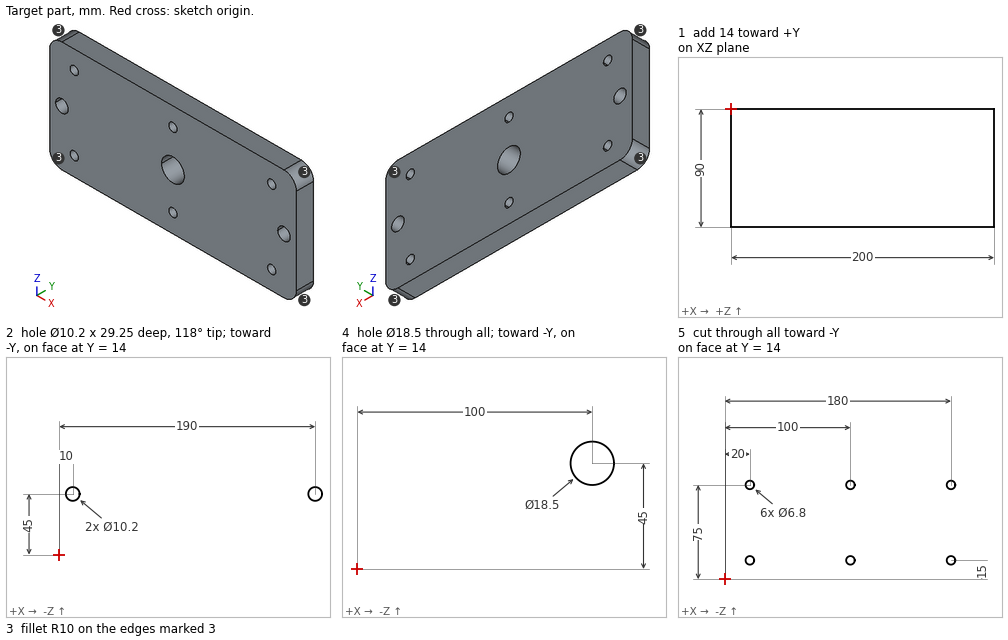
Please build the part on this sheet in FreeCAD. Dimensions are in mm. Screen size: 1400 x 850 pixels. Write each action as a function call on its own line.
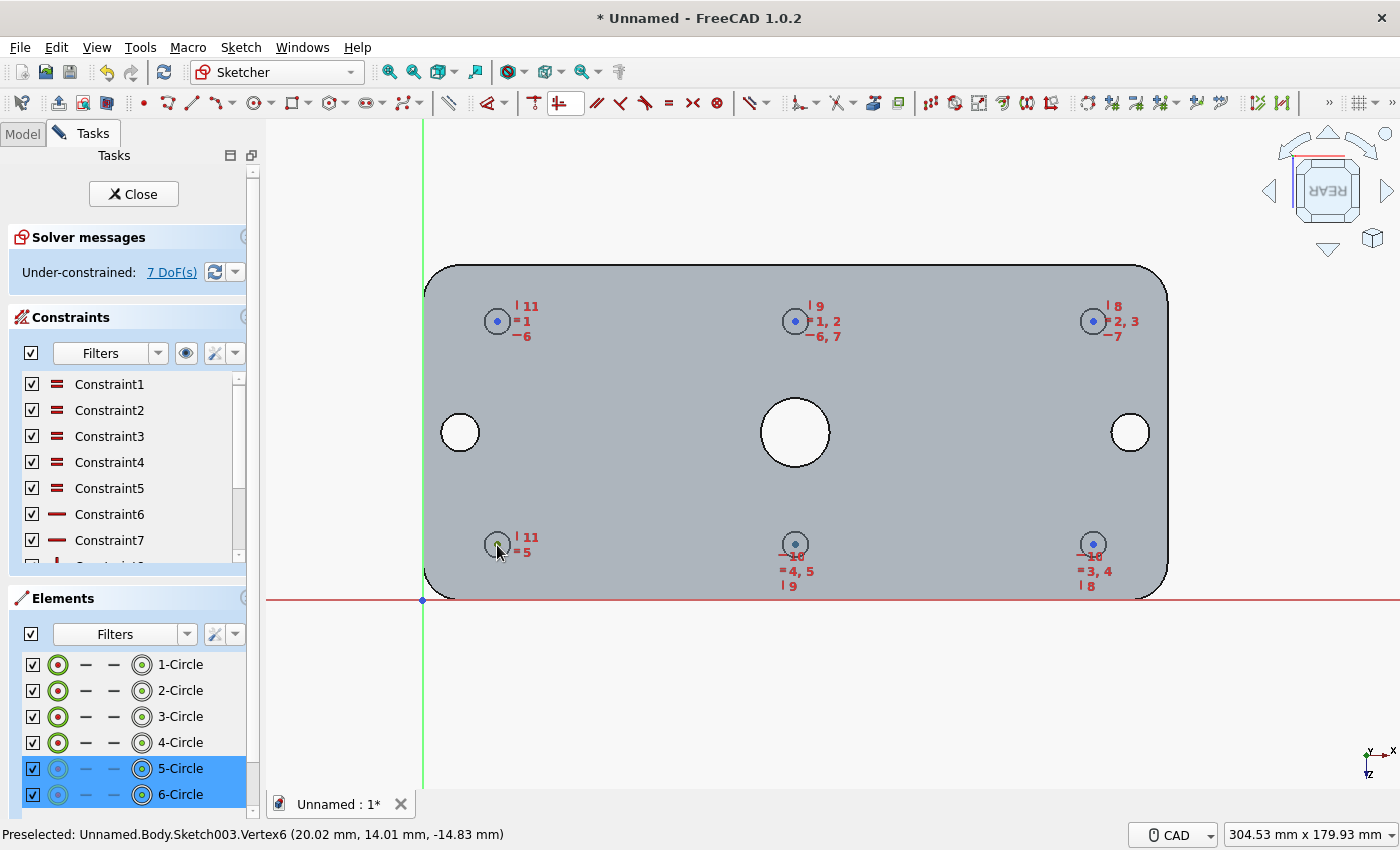
click(578, 104)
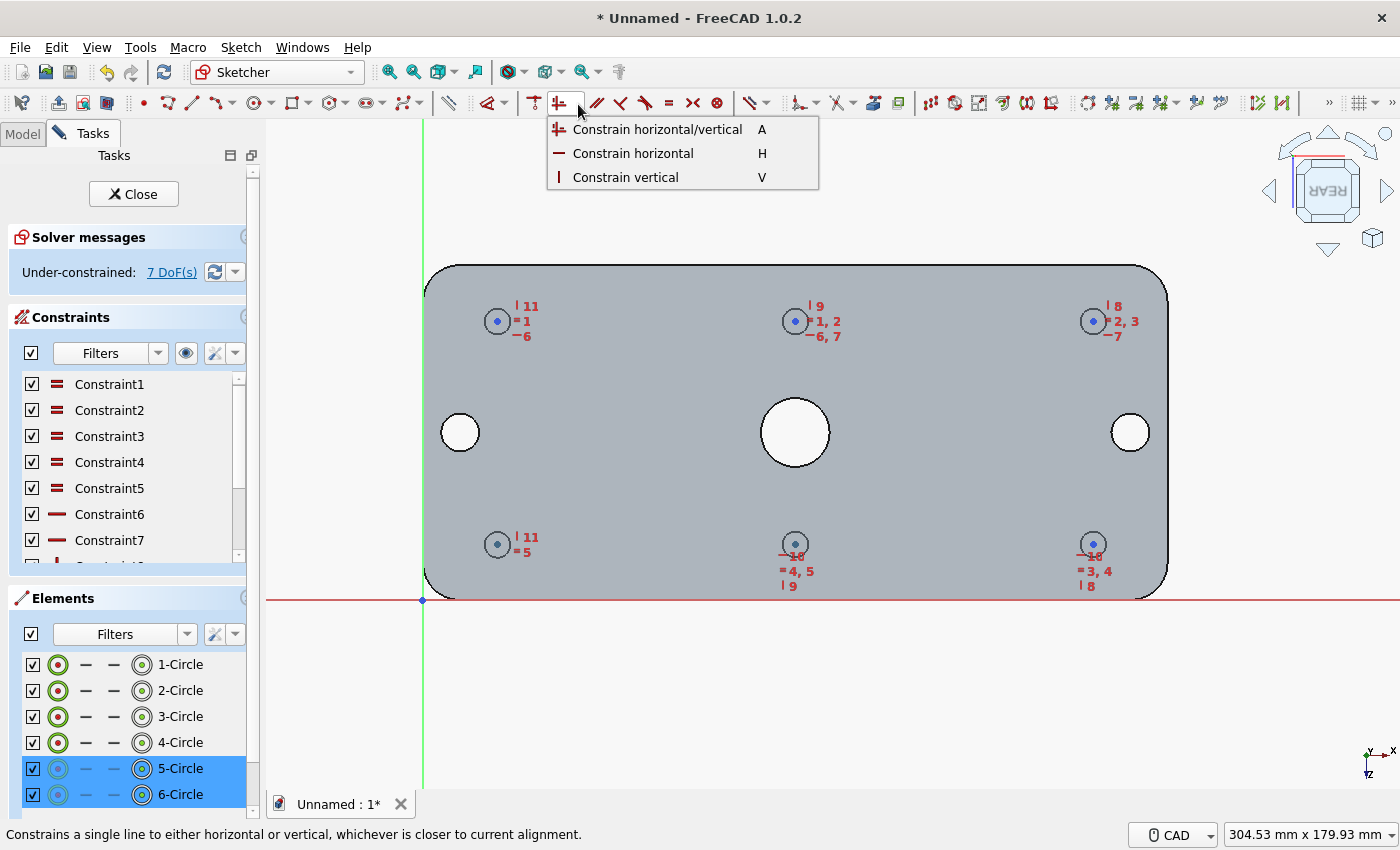
click(683, 153)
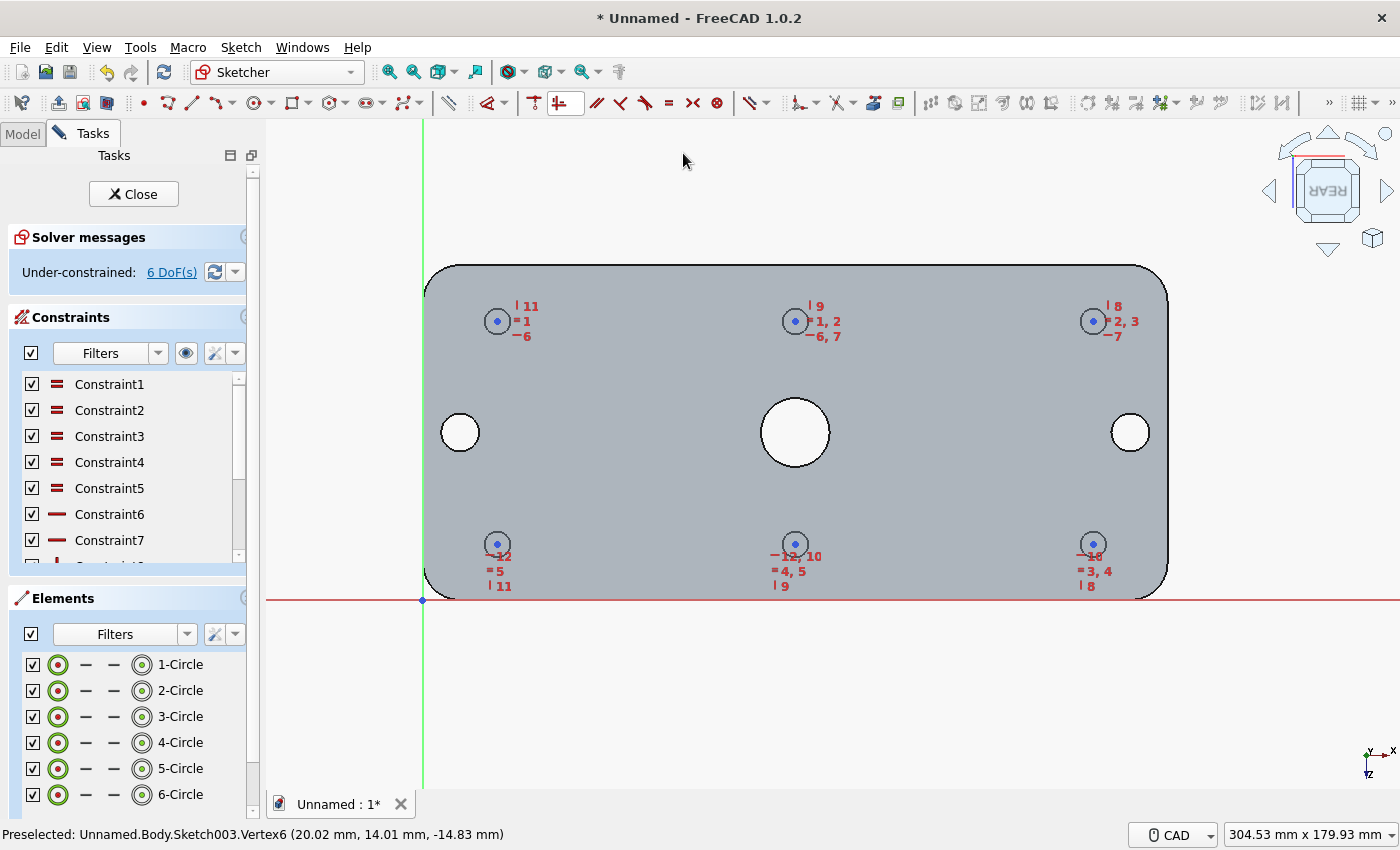
key(d)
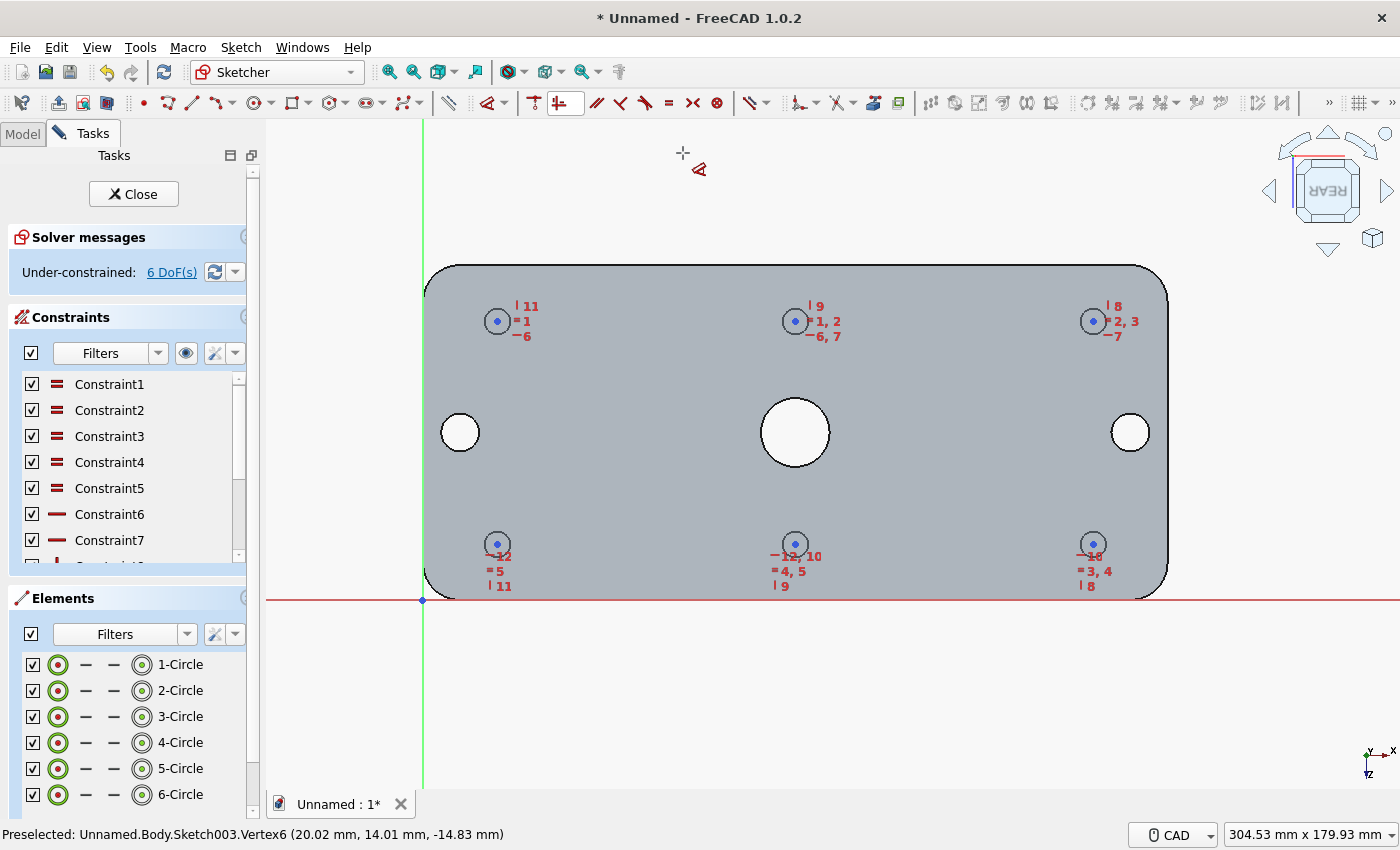
scroll(506, 313, up, 3)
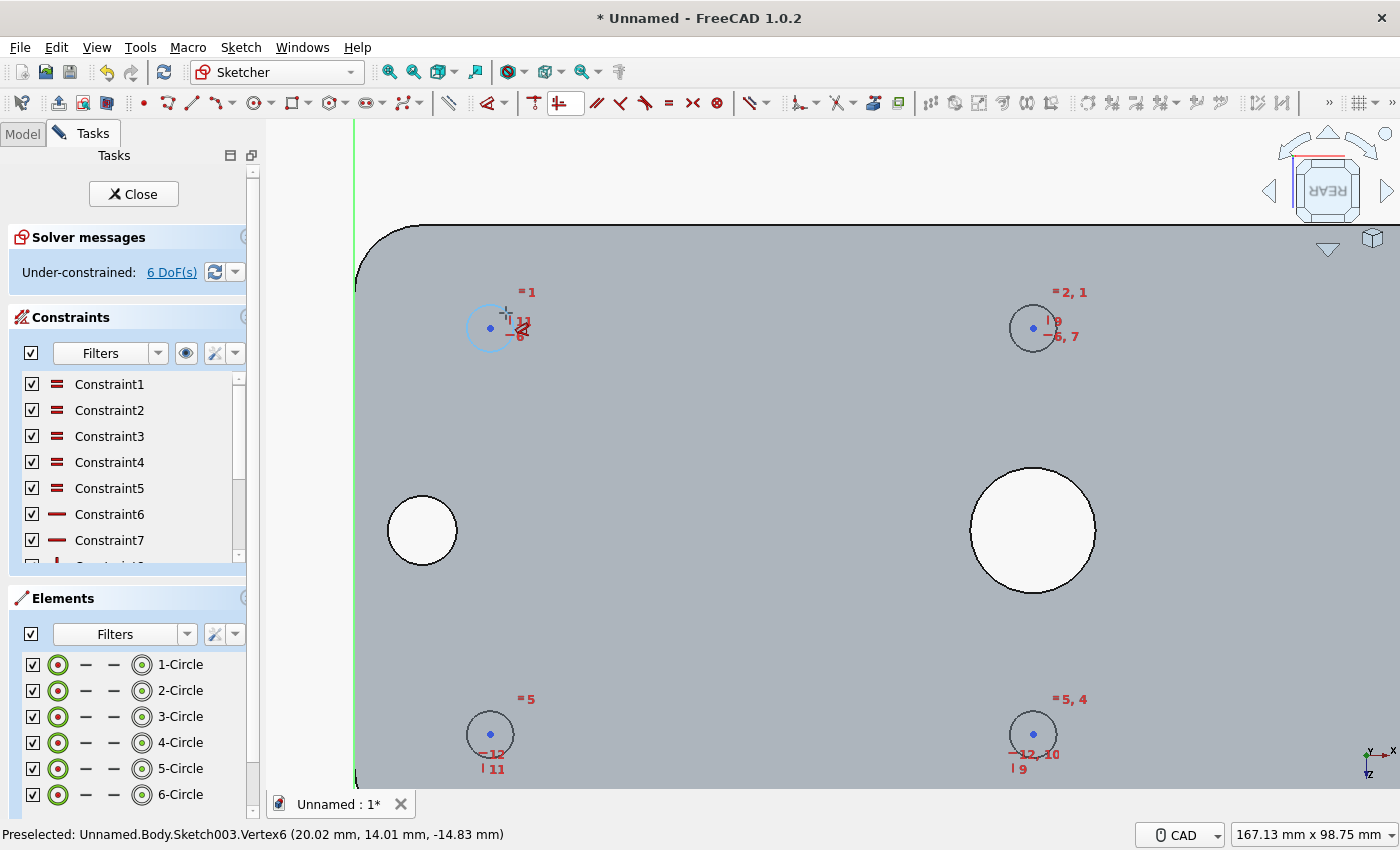
click(507, 312)
click(530, 290)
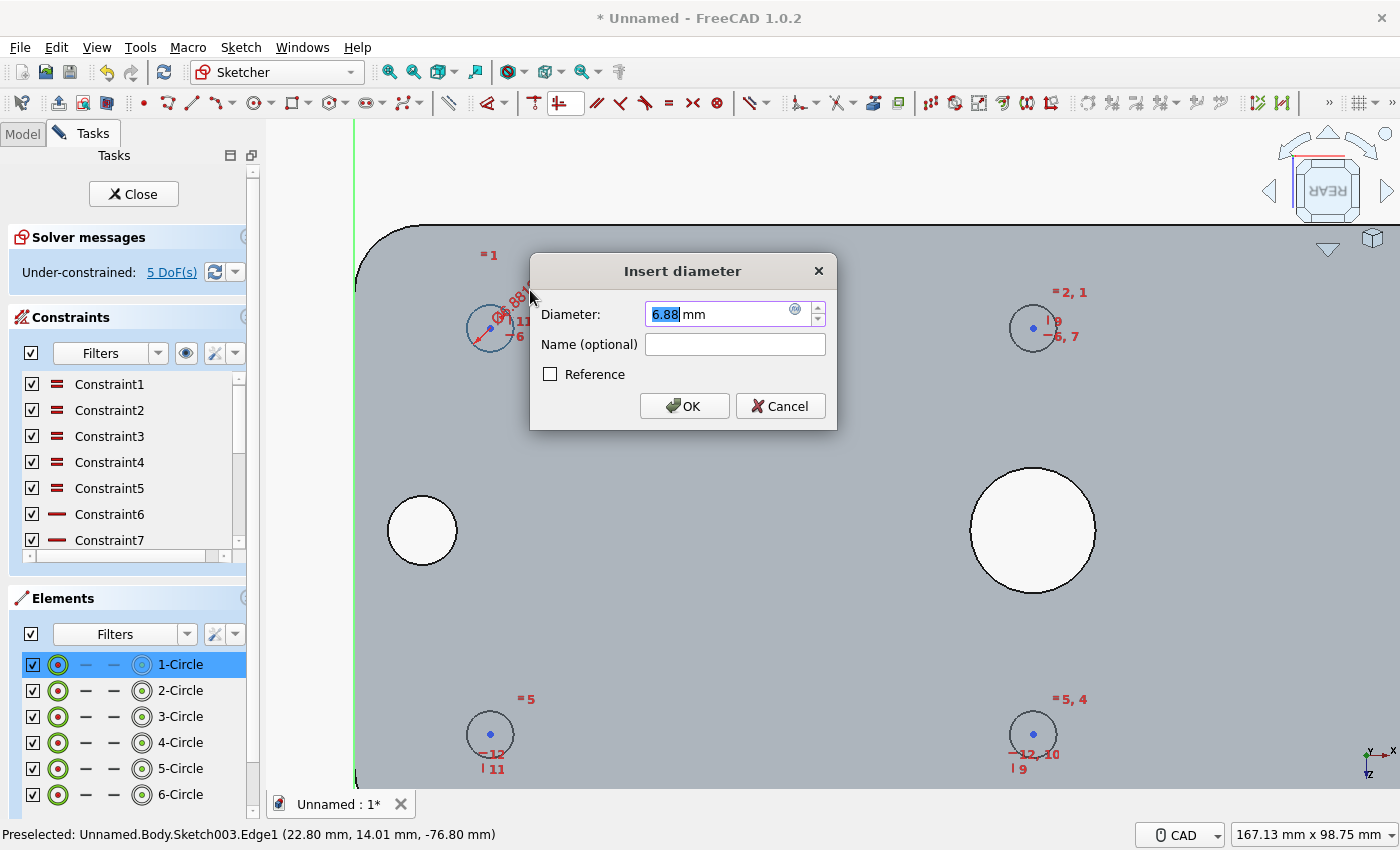
text(6.8)
key(Return)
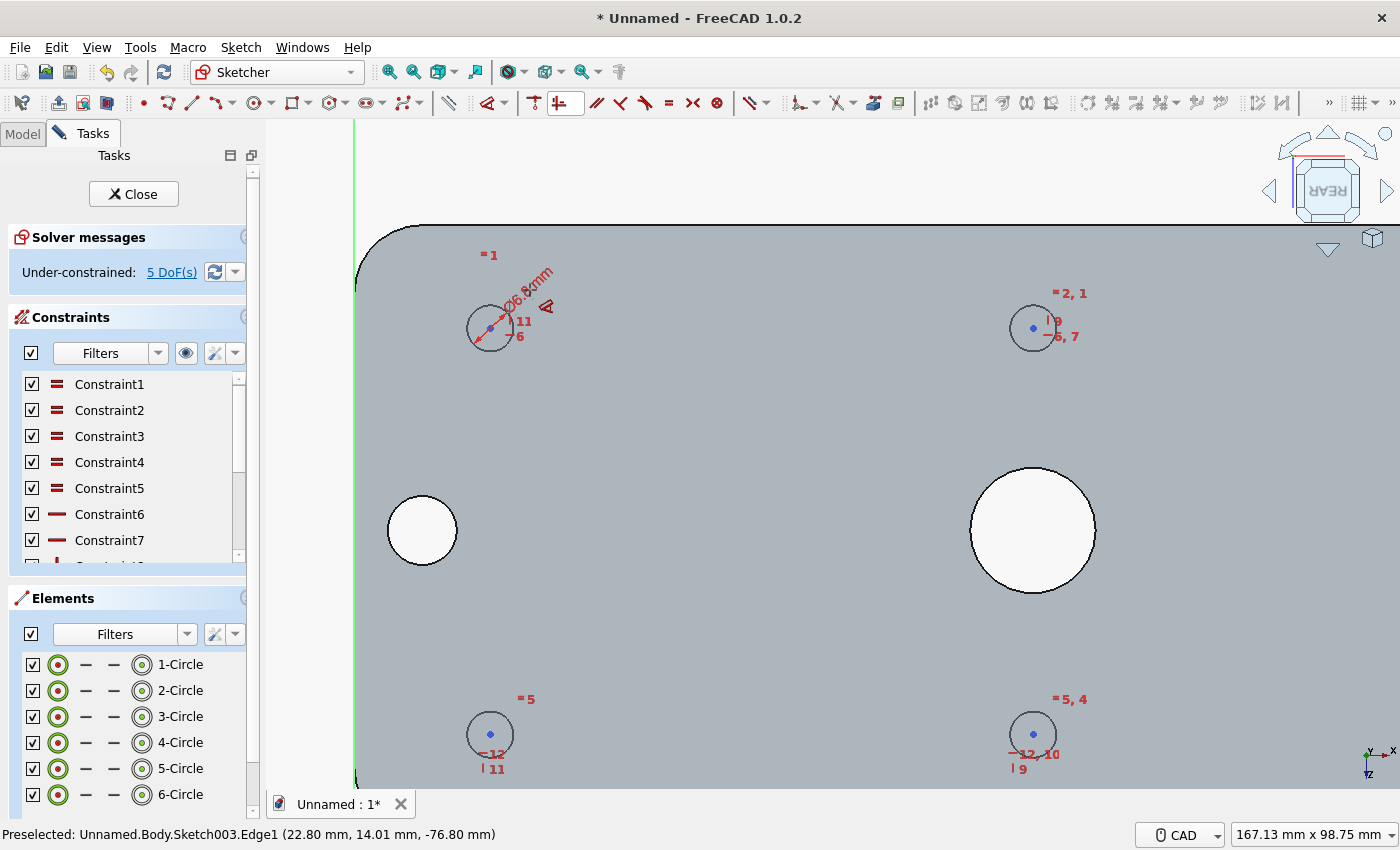
click(490, 328)
click(422, 294)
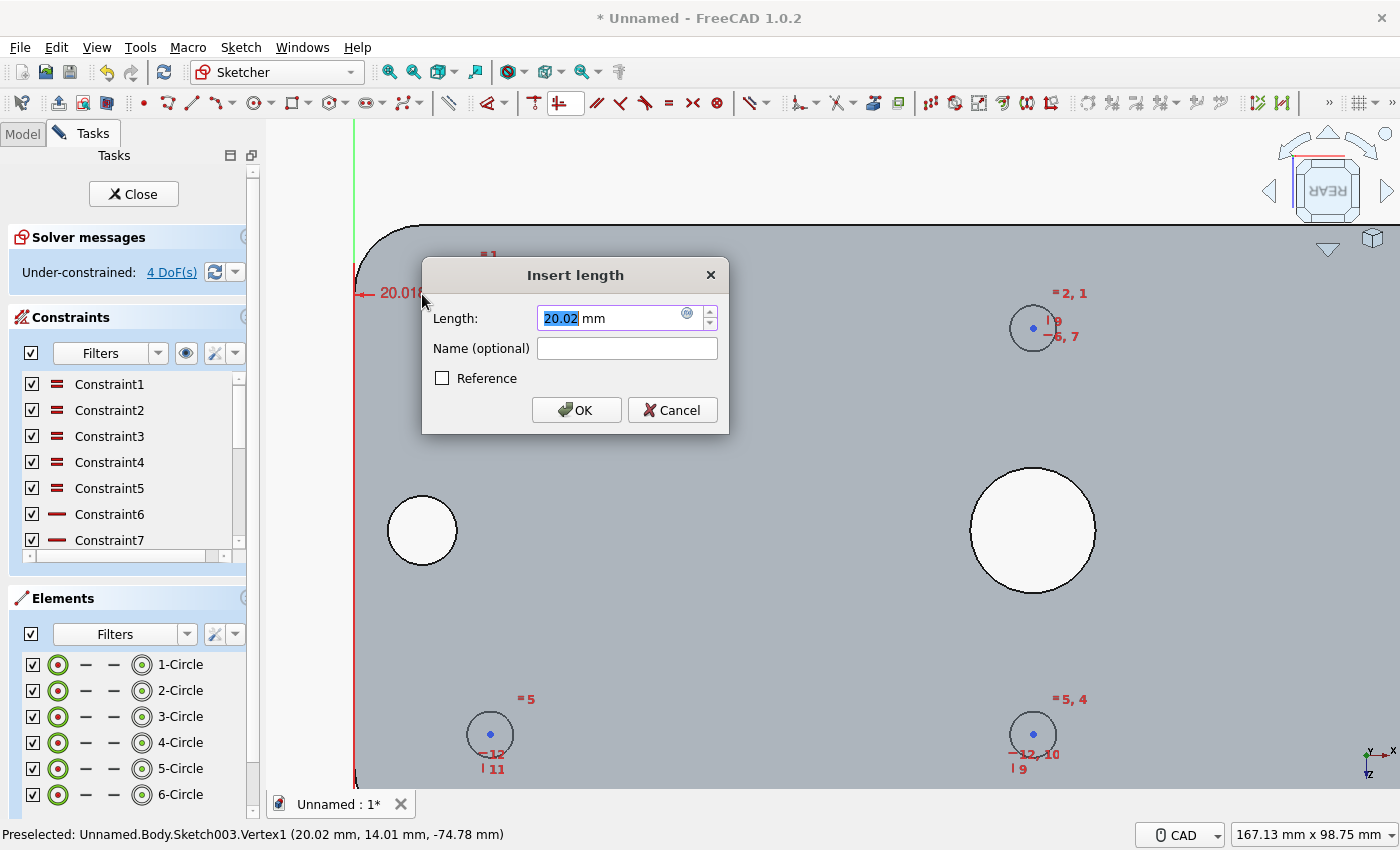
text(20)
key(Return)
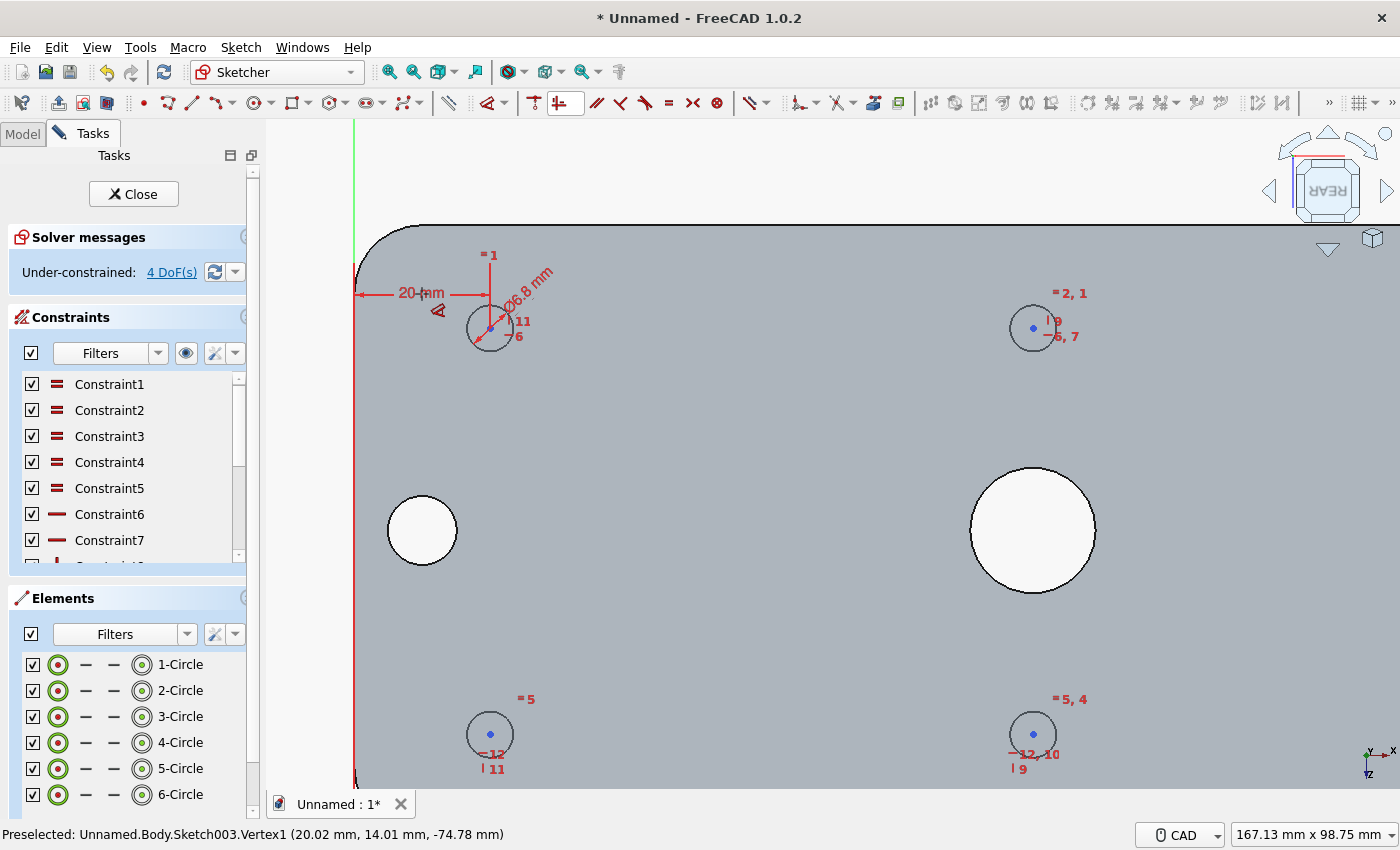
click(490, 328)
click(320, 545)